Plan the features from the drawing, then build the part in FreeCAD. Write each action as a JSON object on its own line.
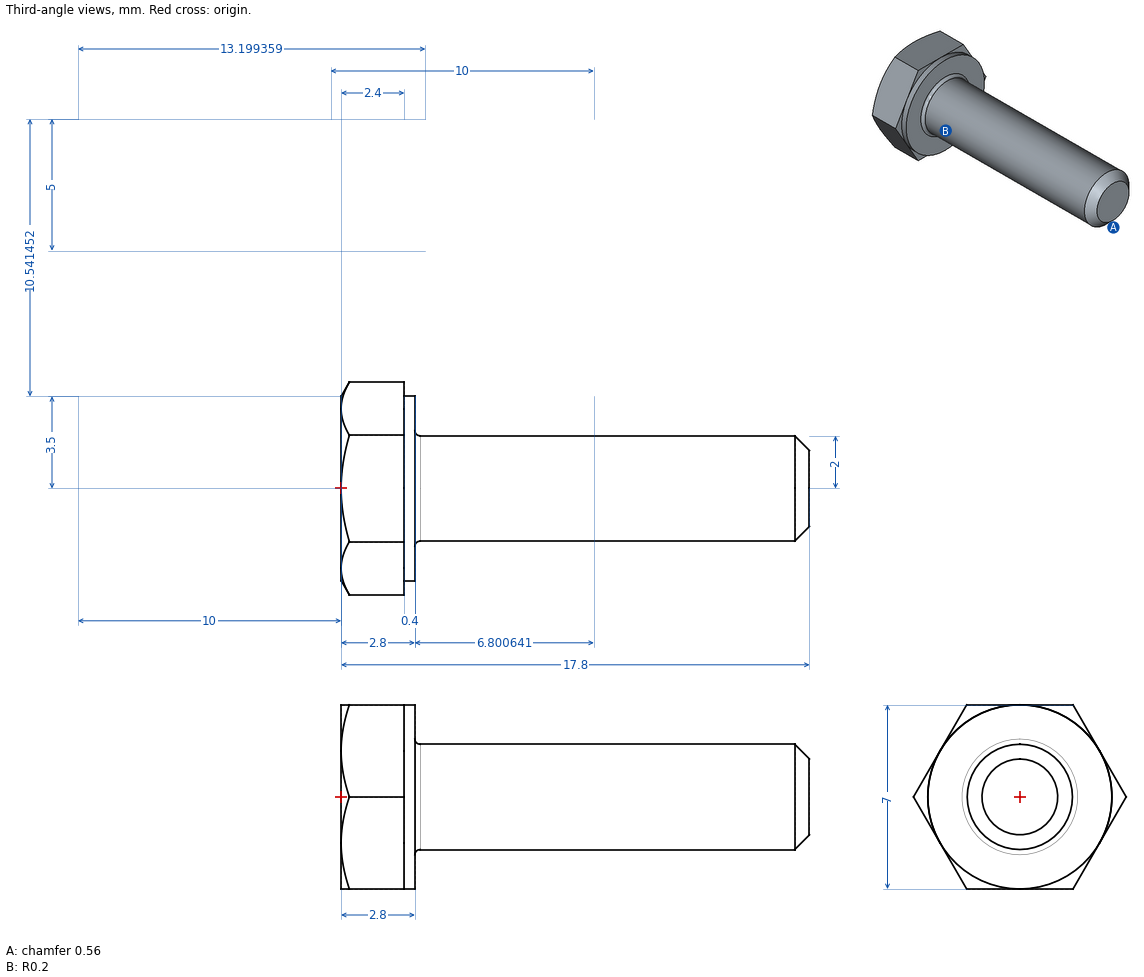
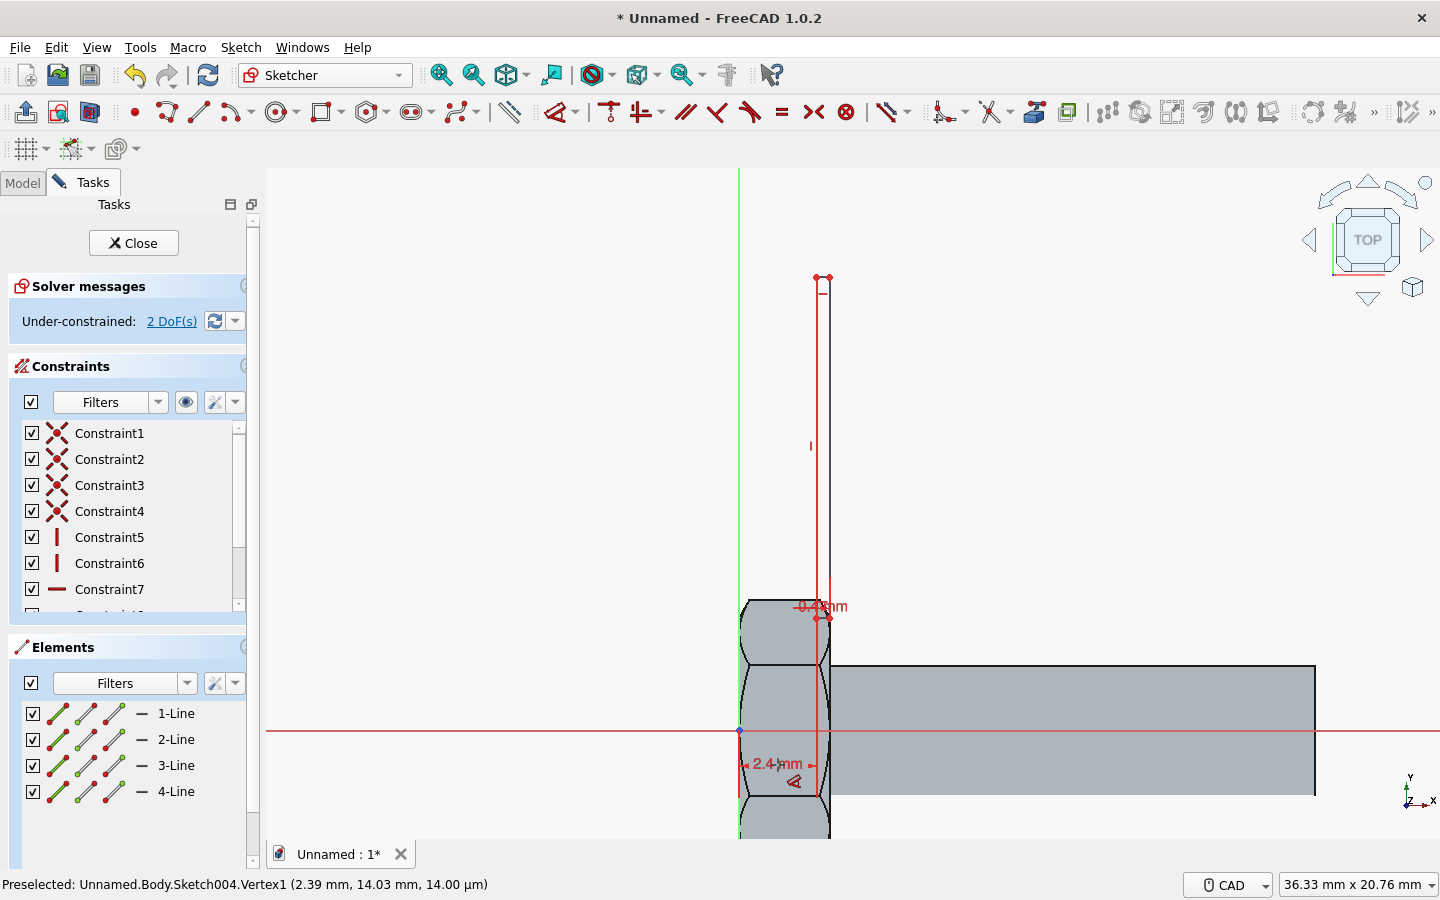
{"action": "left_click", "coordinate": [817, 618]}
{"action": "left_click", "coordinate": [705, 674]}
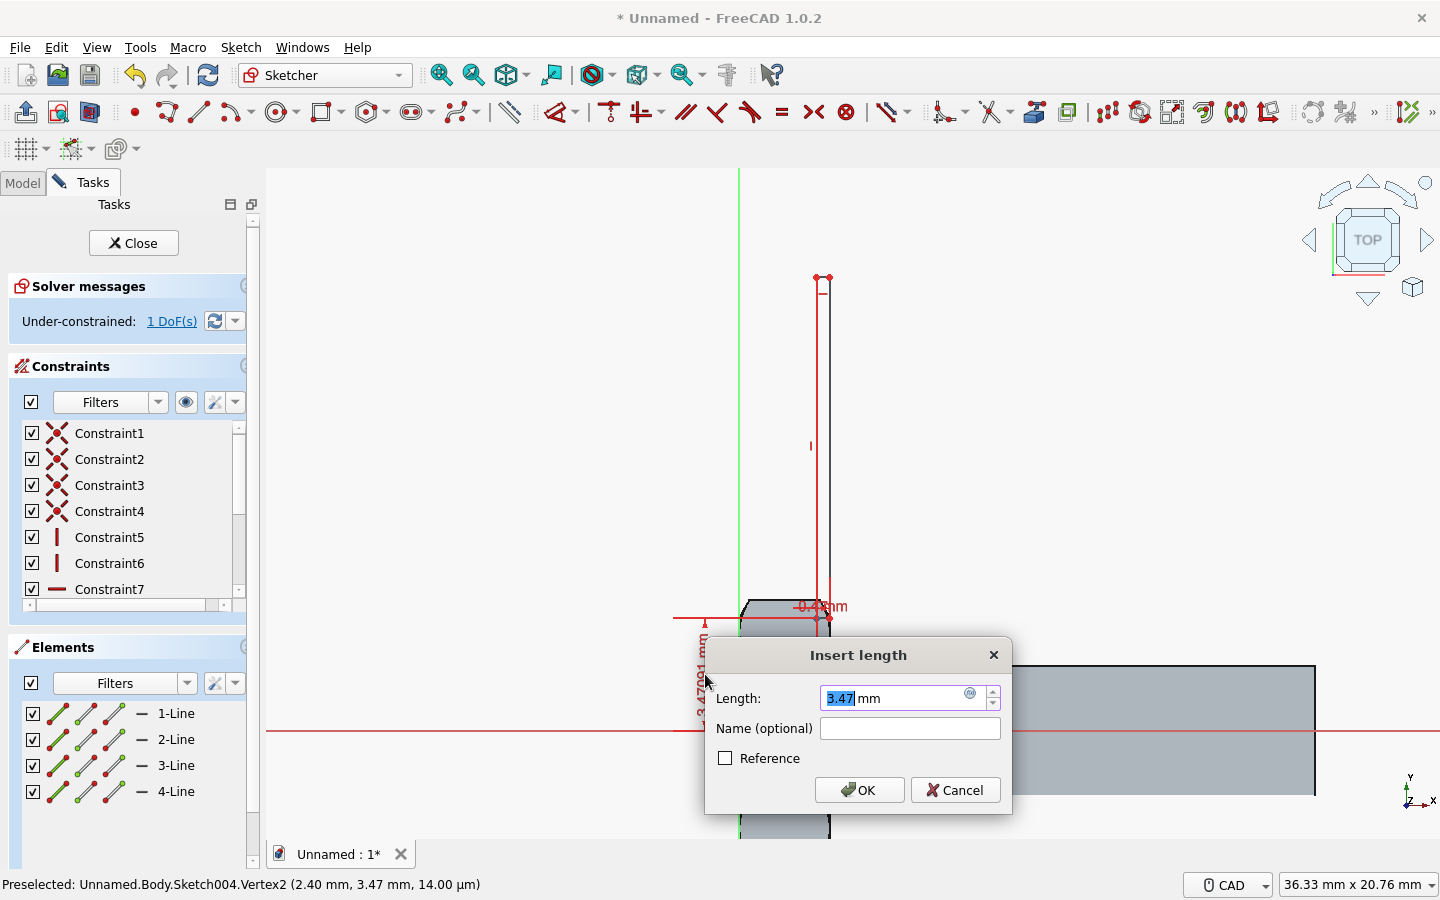
{"action": "type", "text": "3.5"}
{"action": "key", "text": "Return"}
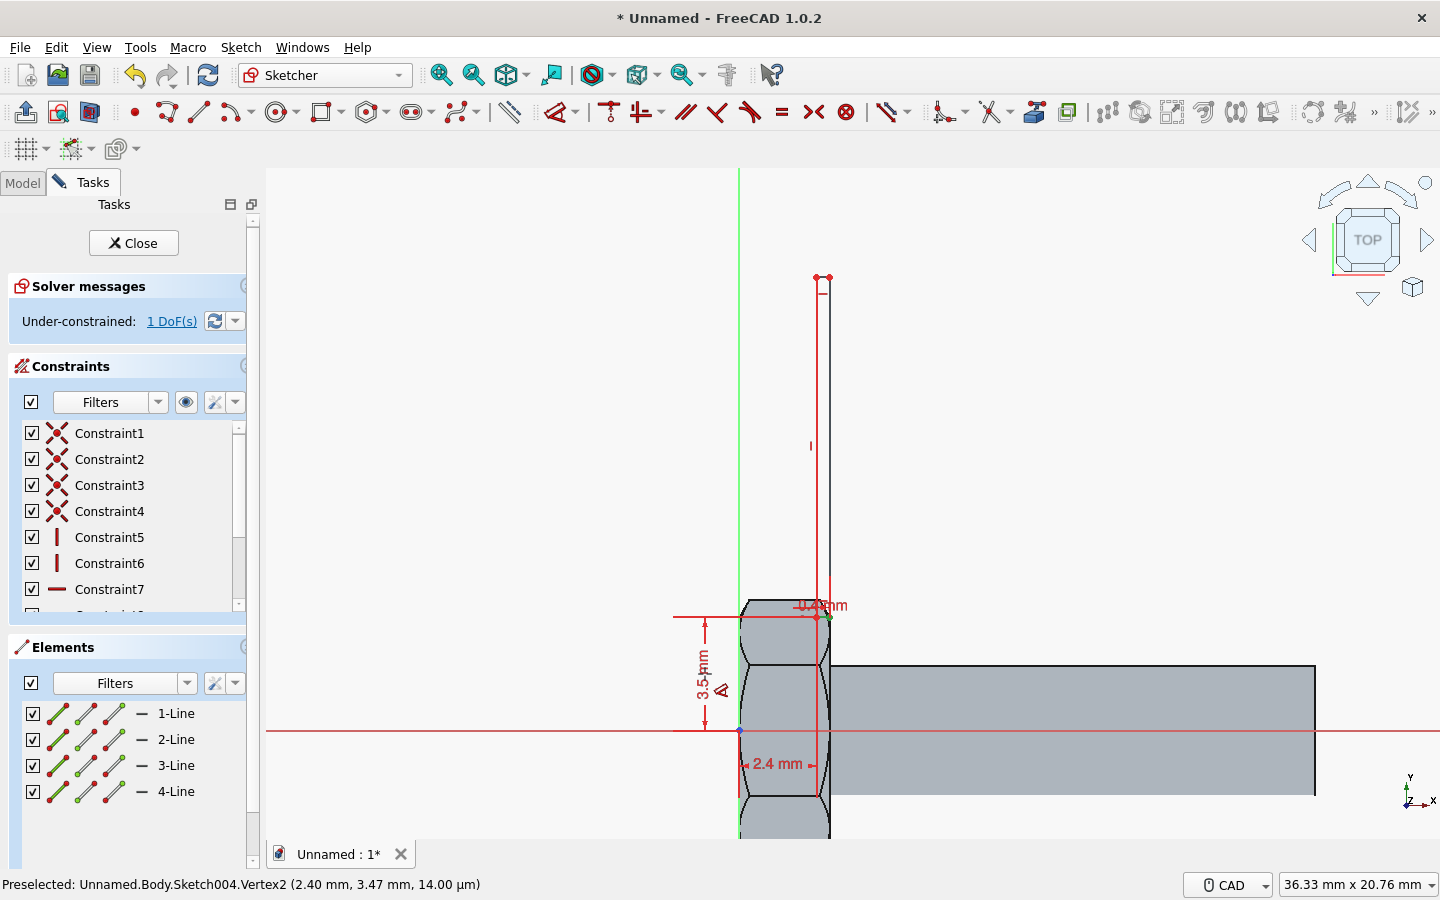
{"action": "left_click", "coordinate": [817, 379]}
{"action": "left_click", "coordinate": [851, 447]}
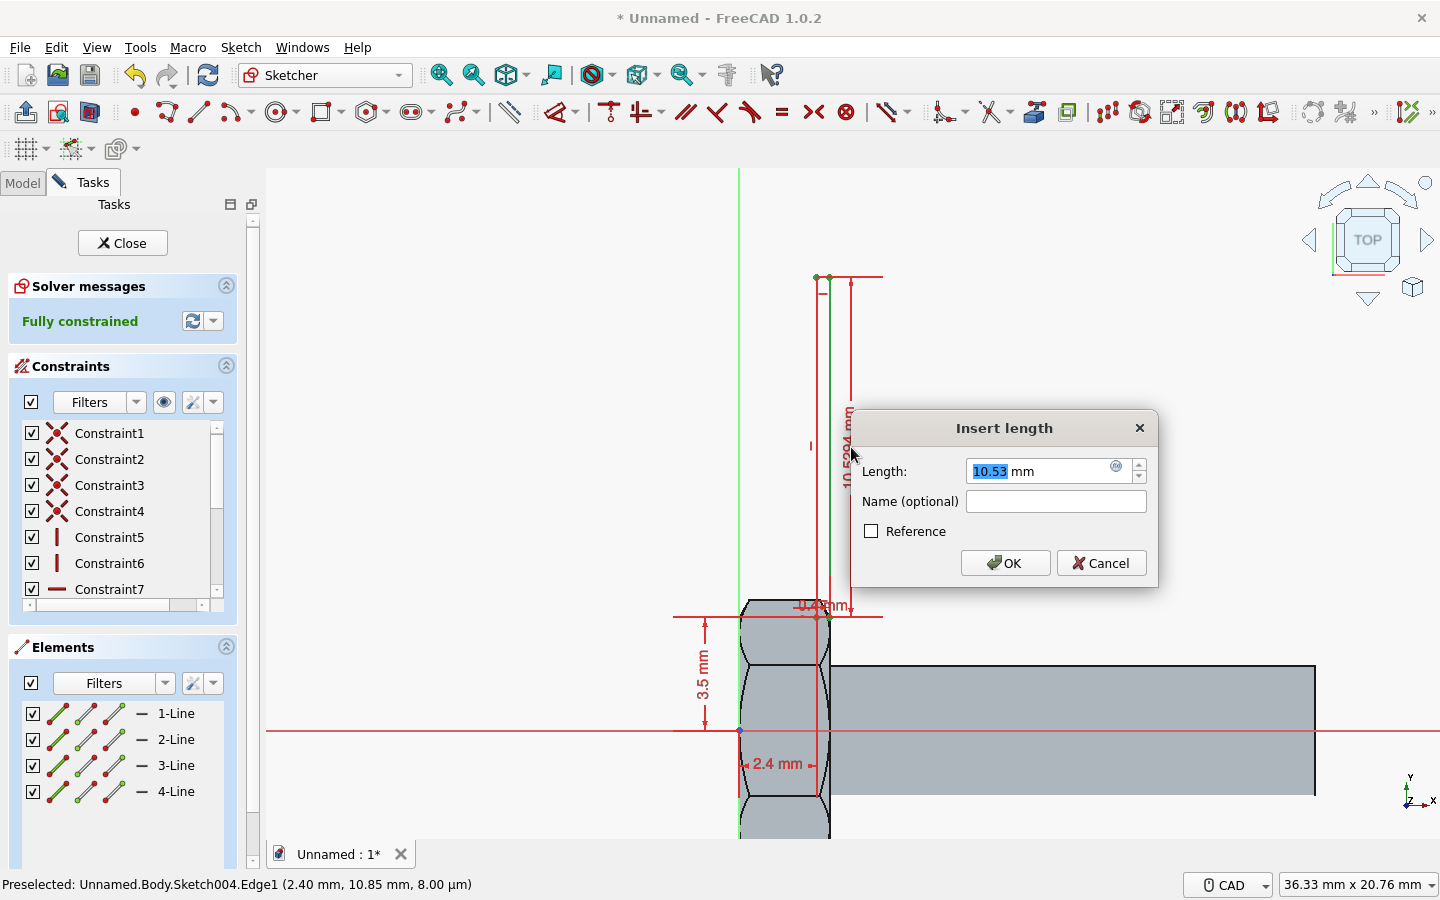
{"action": "type", "text": "10.541452"}
{"action": "key", "text": "Return"}
{"action": "key", "text": "Escape"}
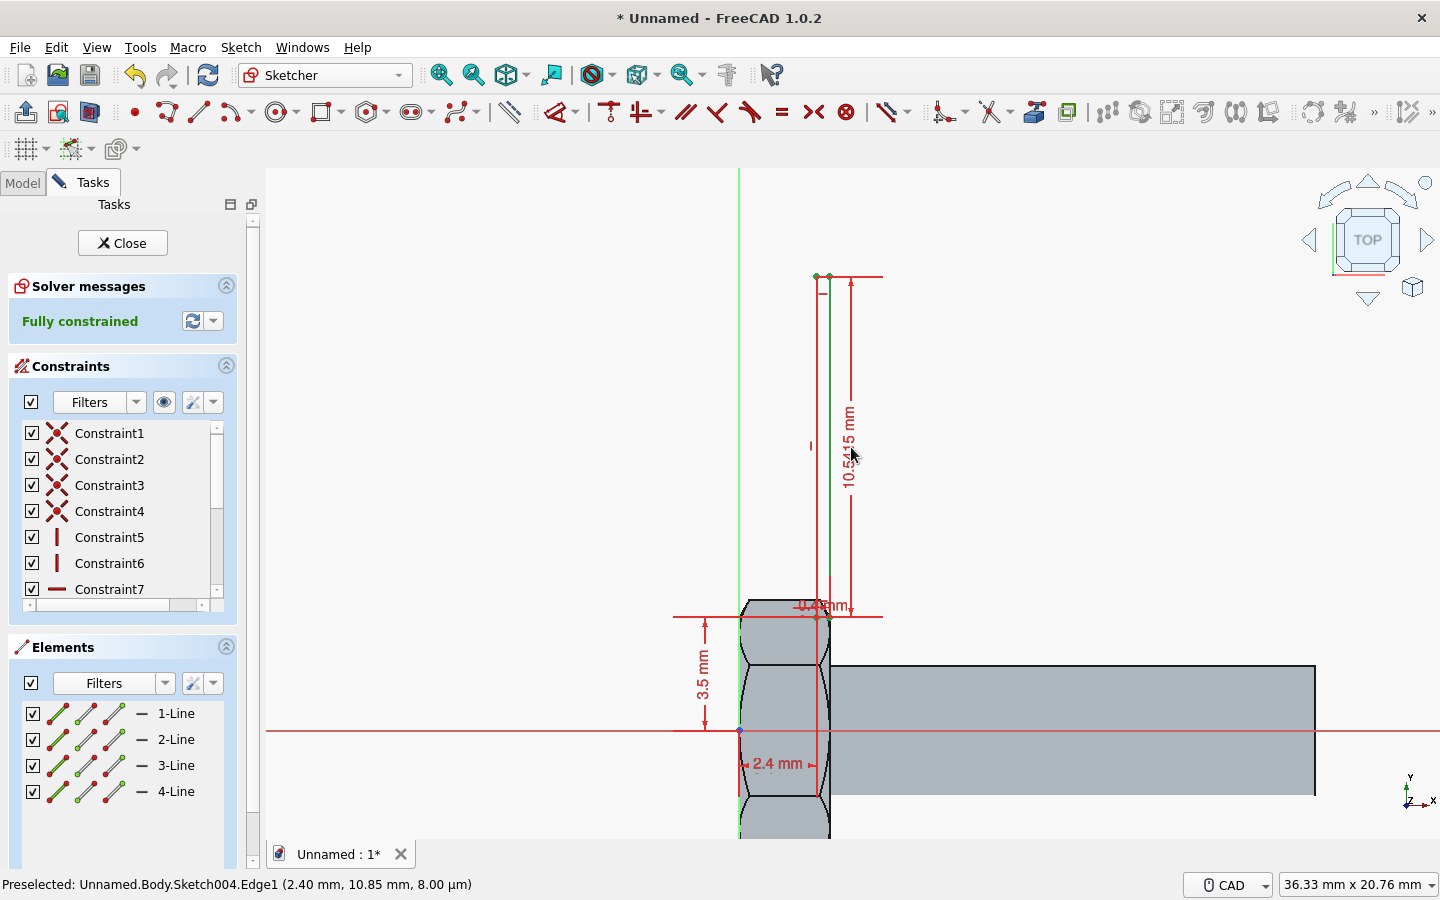
{"action": "left_click", "coordinate": [123, 243]}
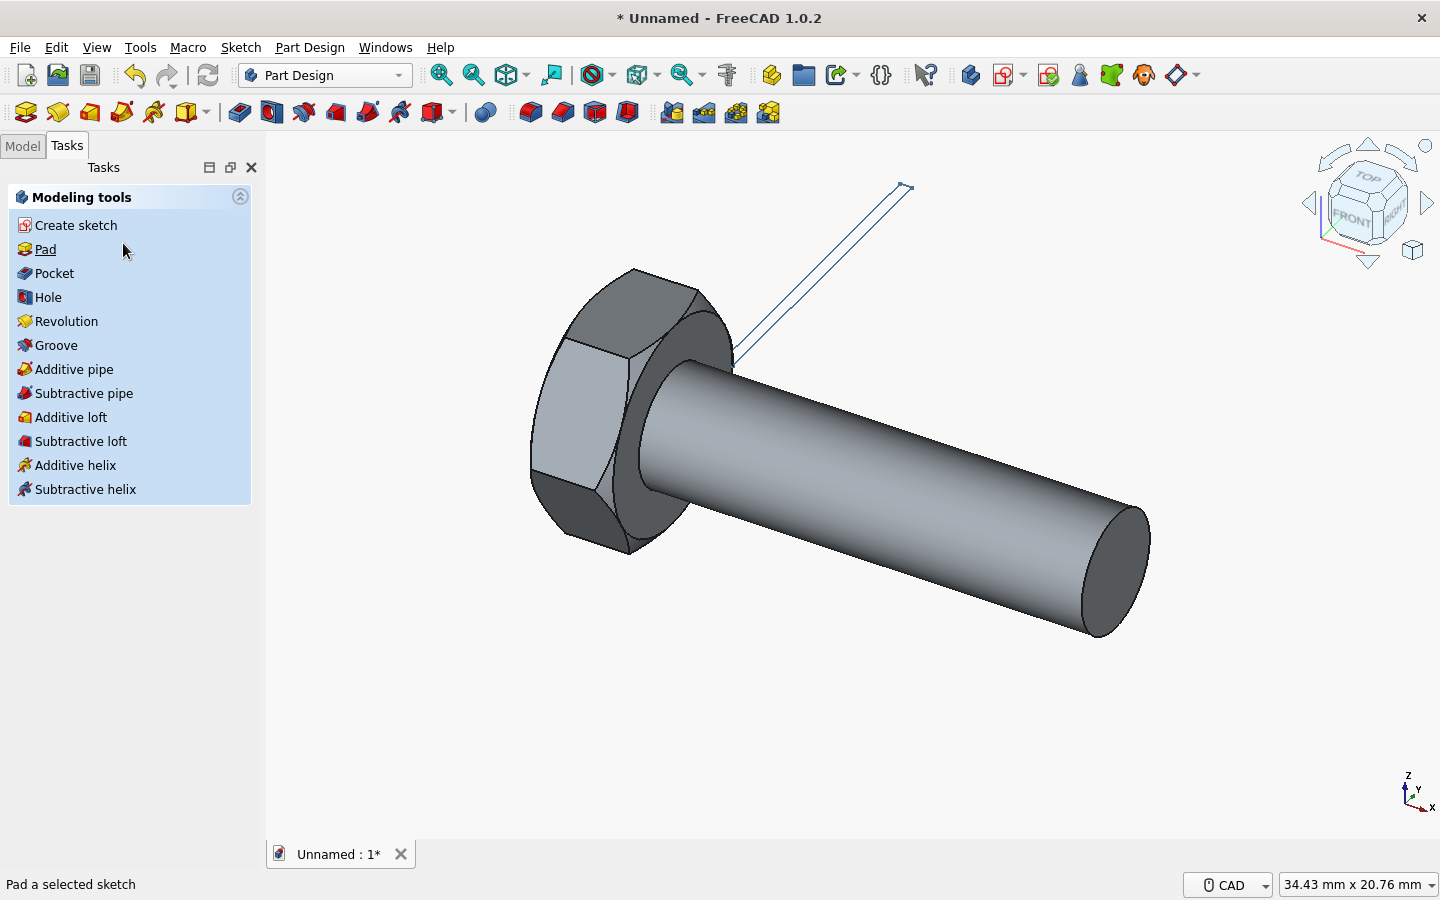
{"action": "left_click", "coordinate": [304, 112]}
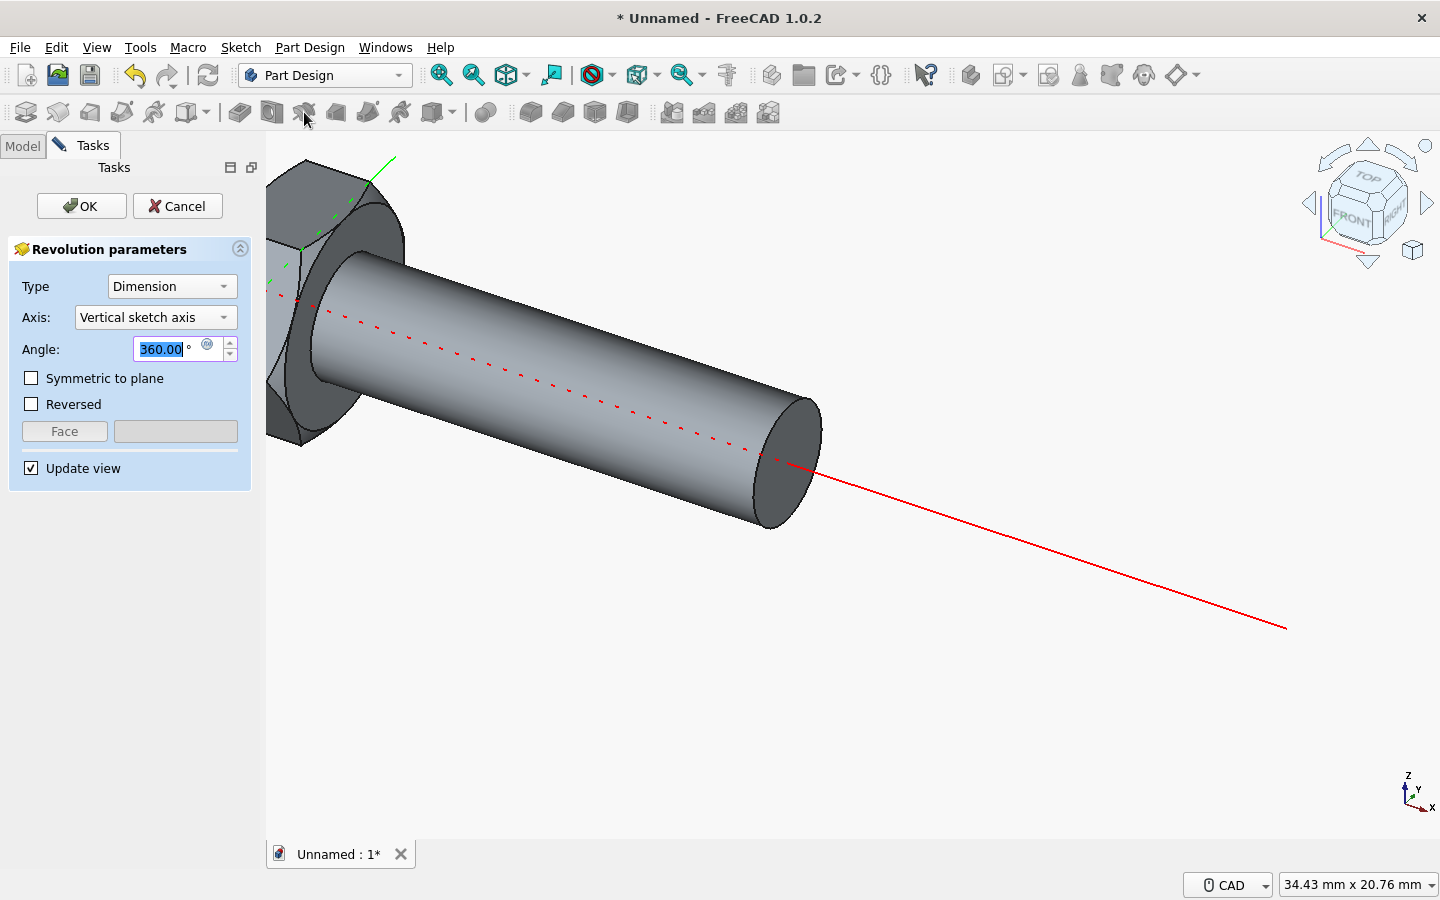
{"action": "left_click", "coordinate": [156, 318]}